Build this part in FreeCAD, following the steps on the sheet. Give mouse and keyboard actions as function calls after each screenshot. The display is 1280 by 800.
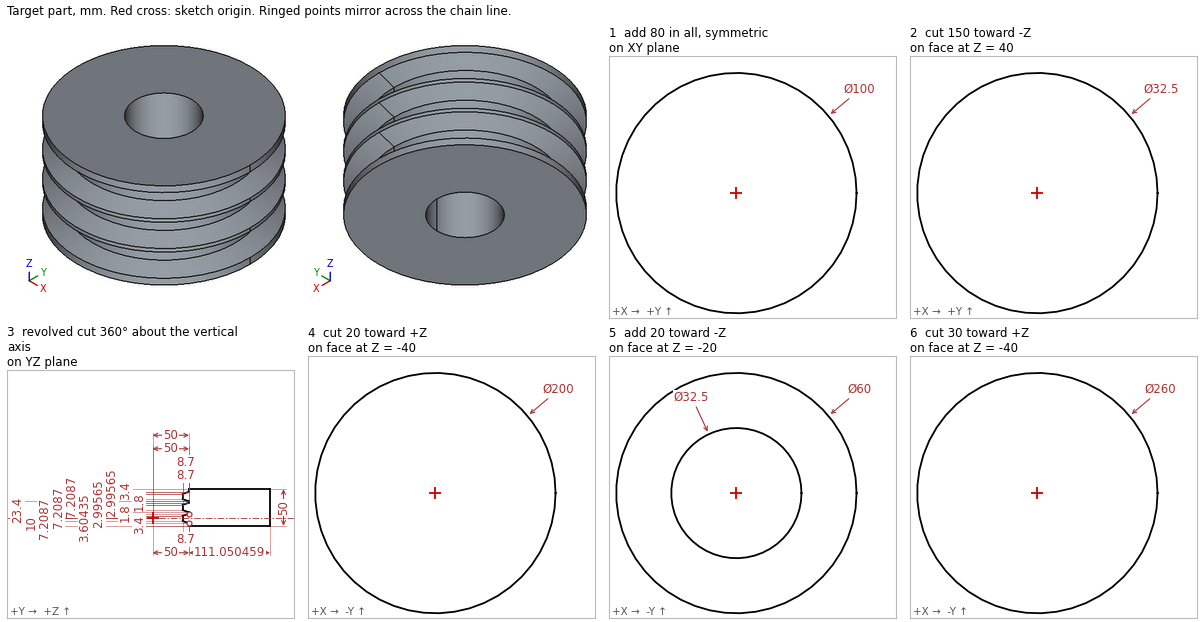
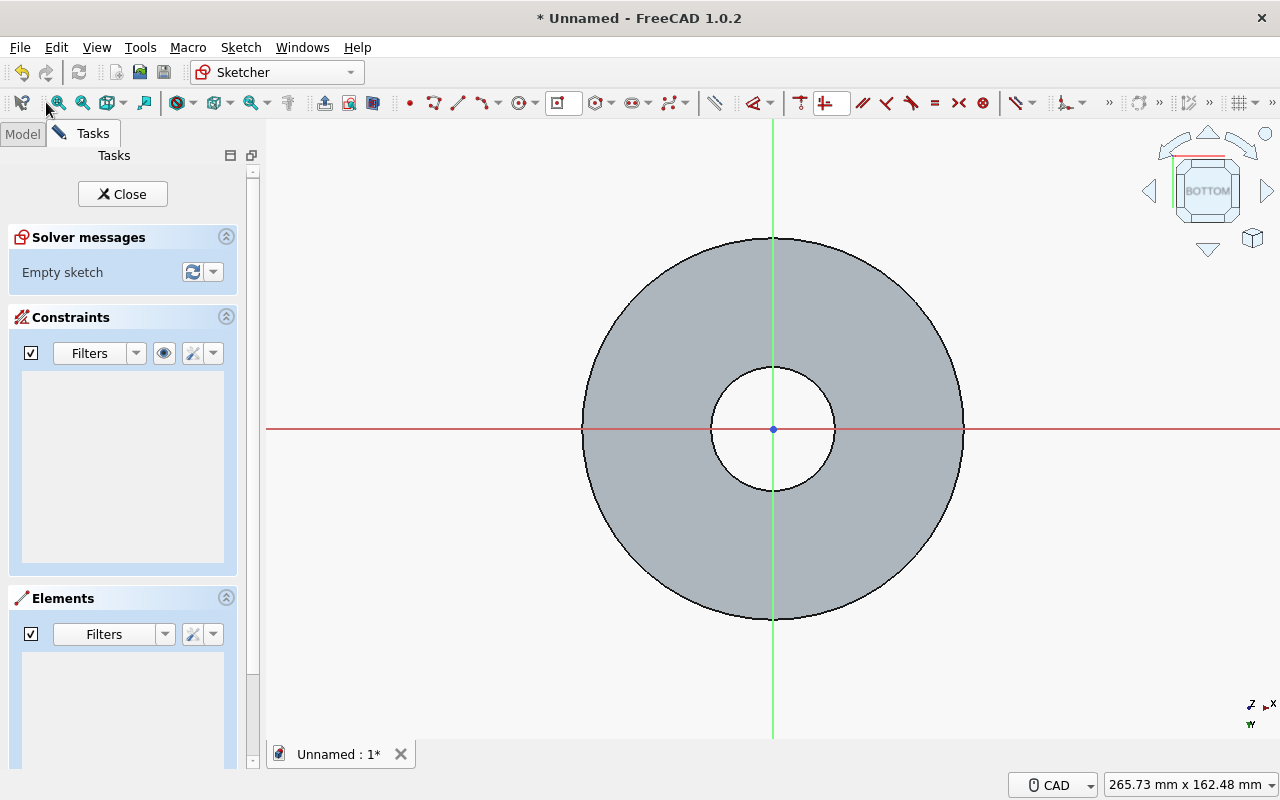
scroll(621, 429, down, 3)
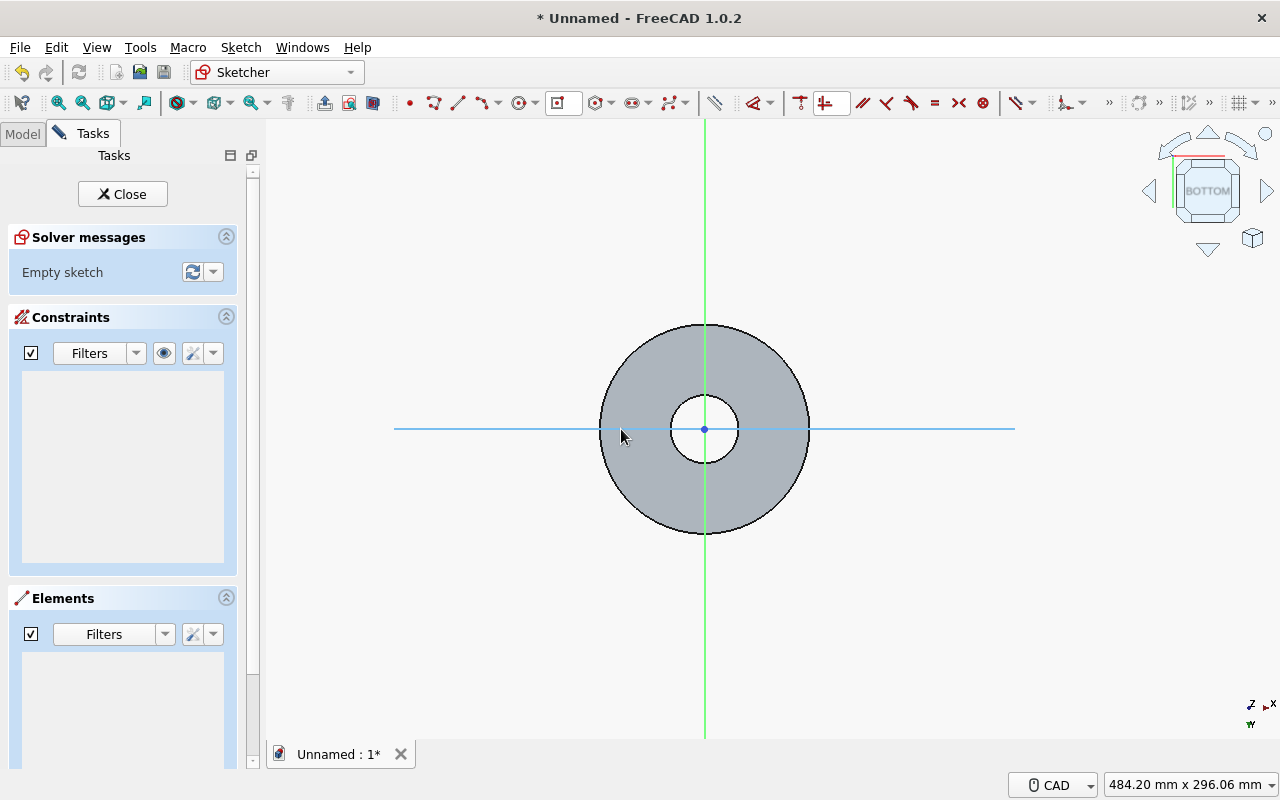
click(520, 104)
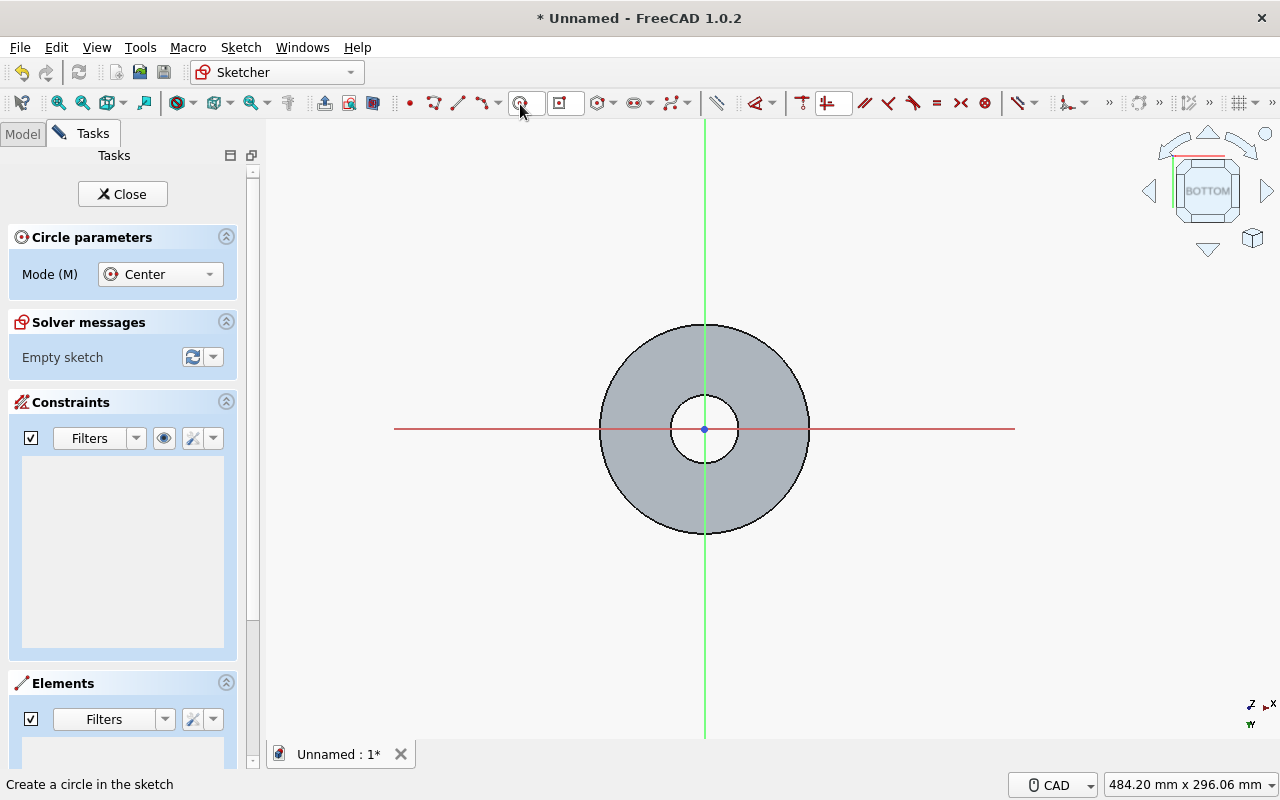
click(705, 429)
click(853, 281)
key(Escape)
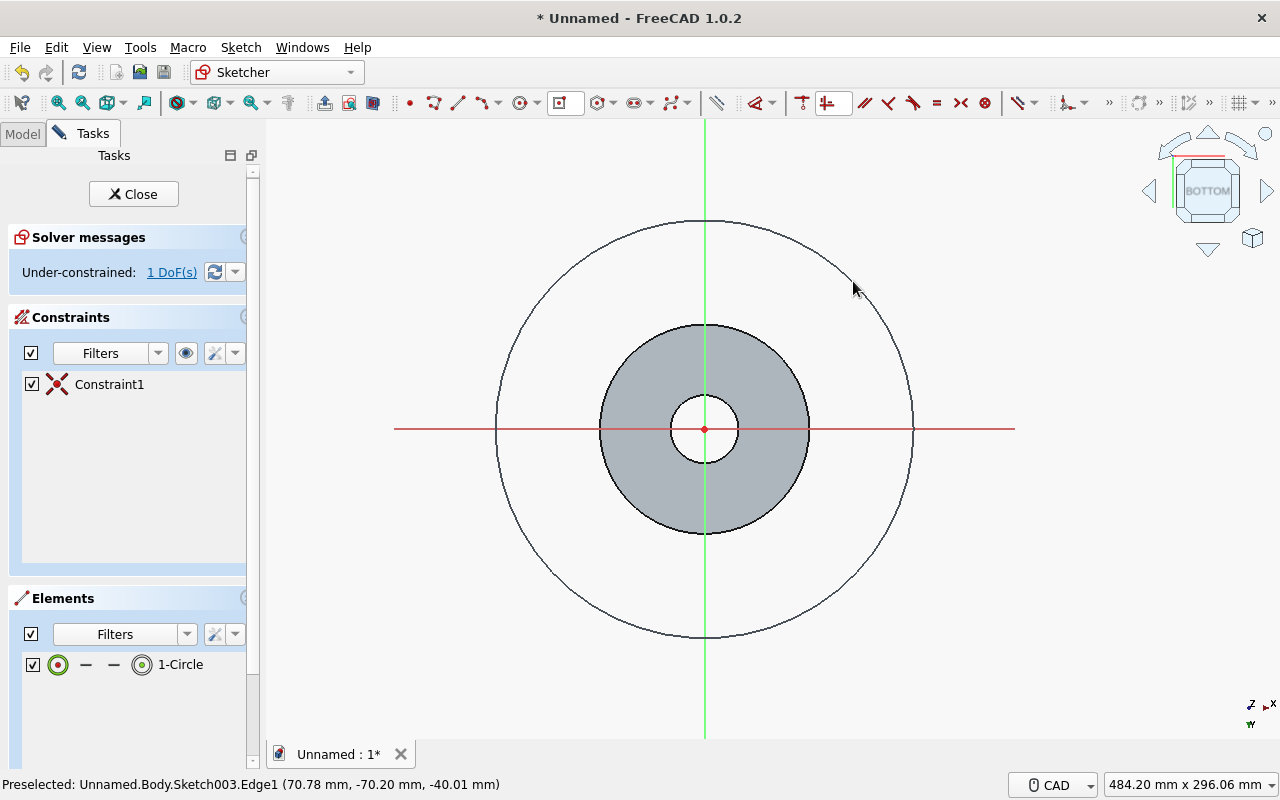
click(756, 104)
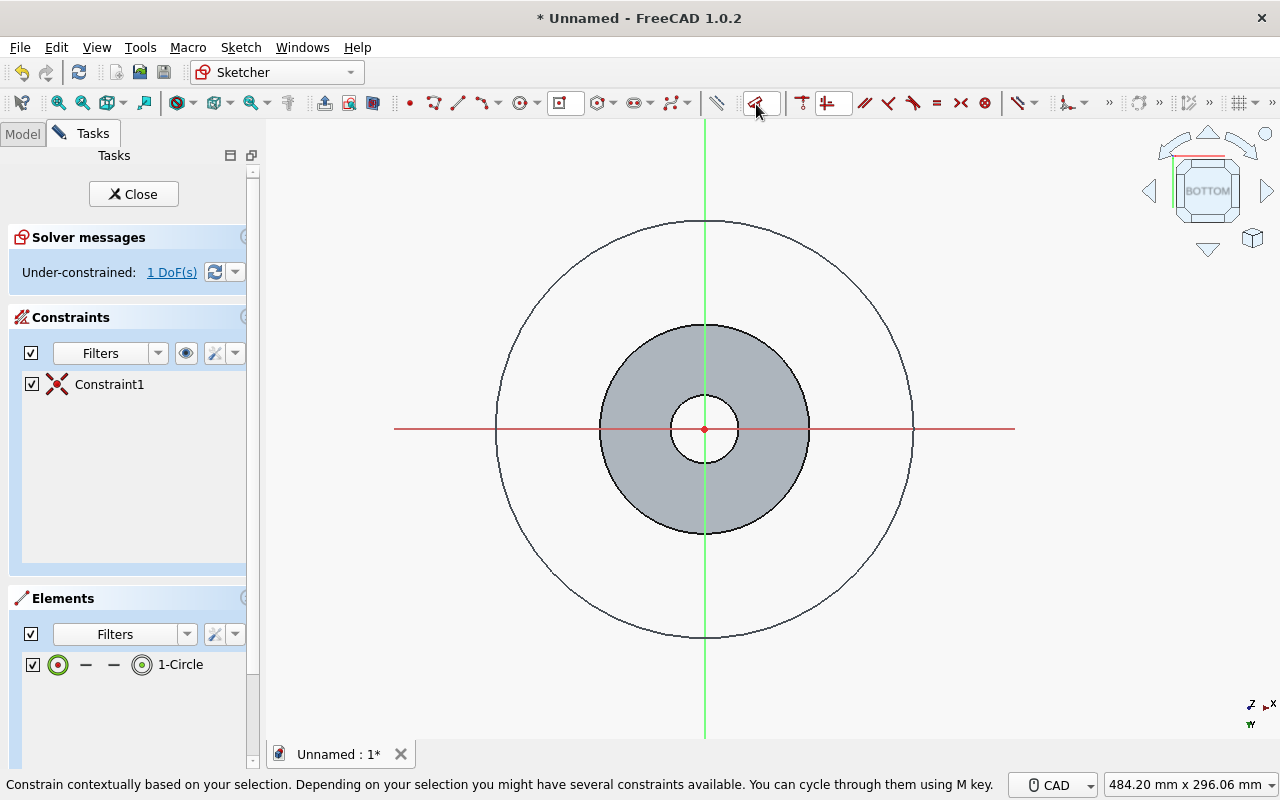
click(852, 281)
click(875, 258)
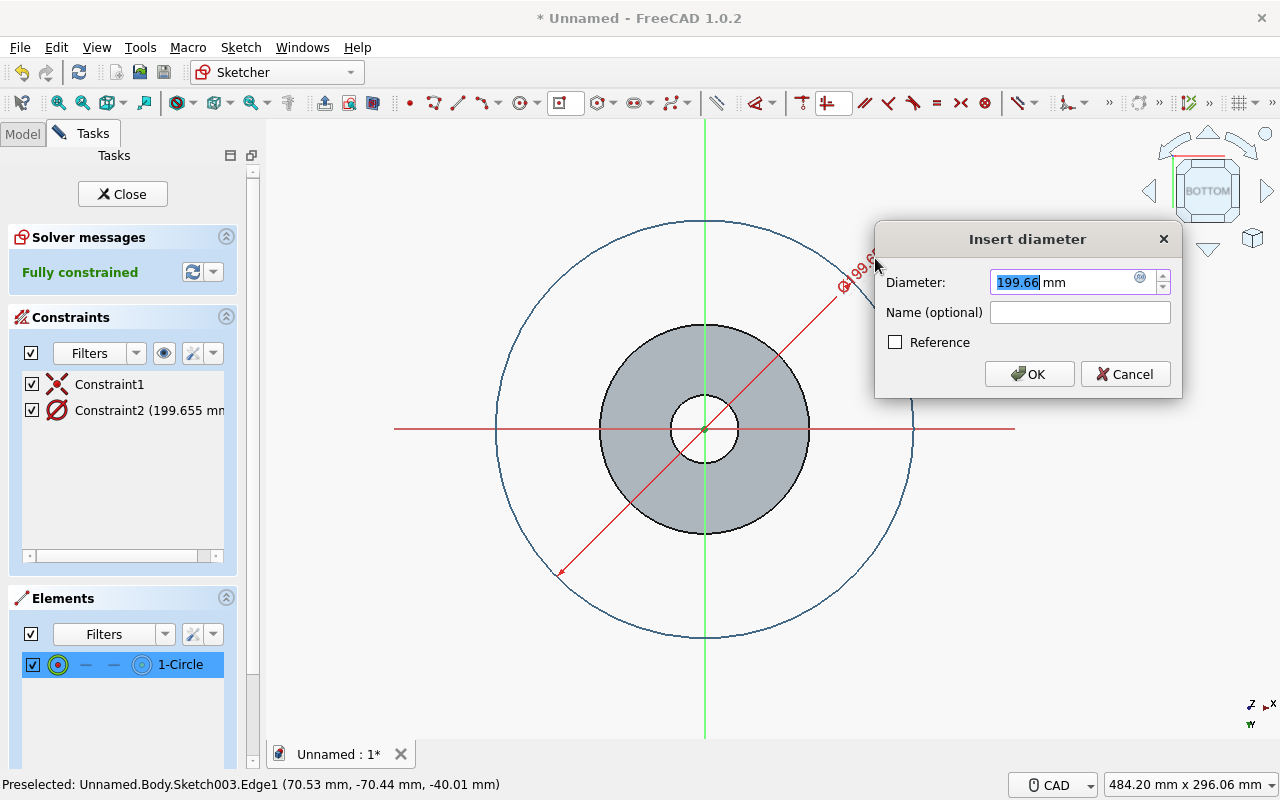
text(200)
key(Return)
key(Escape)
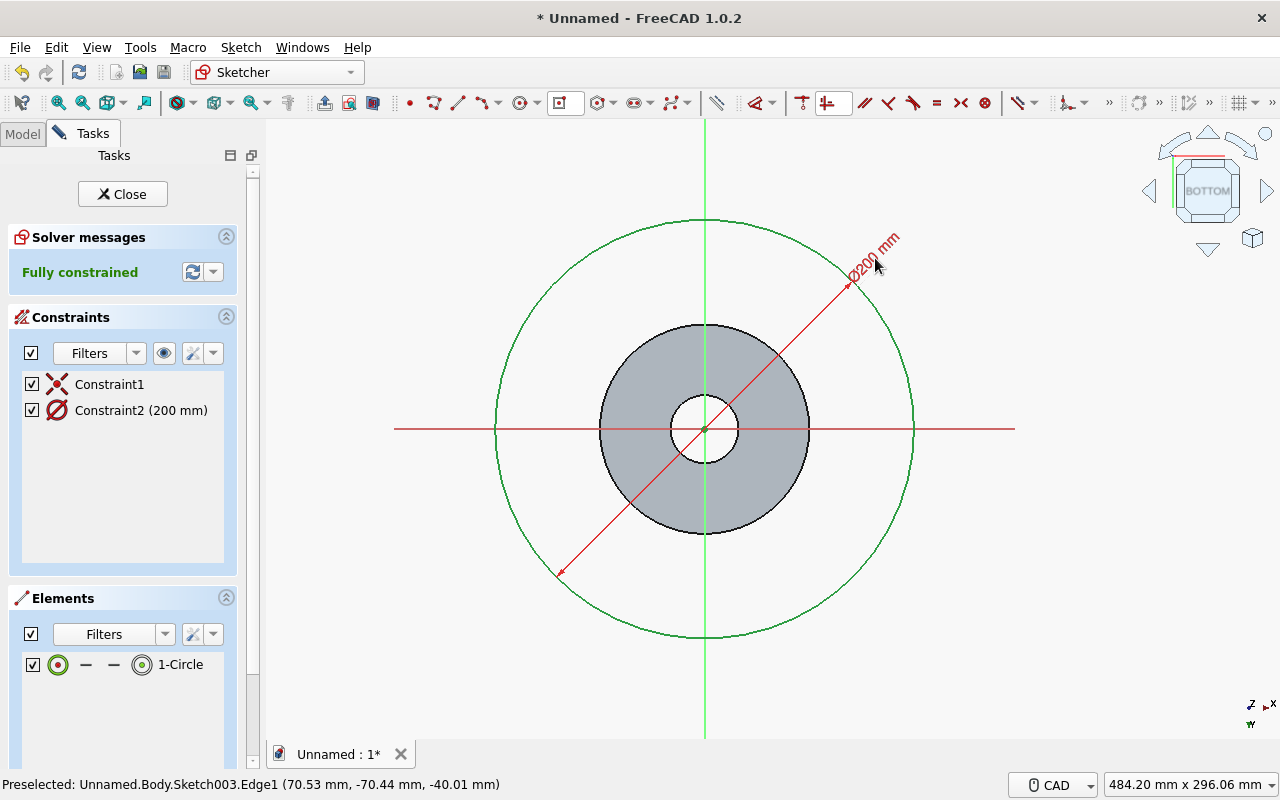
click(123, 194)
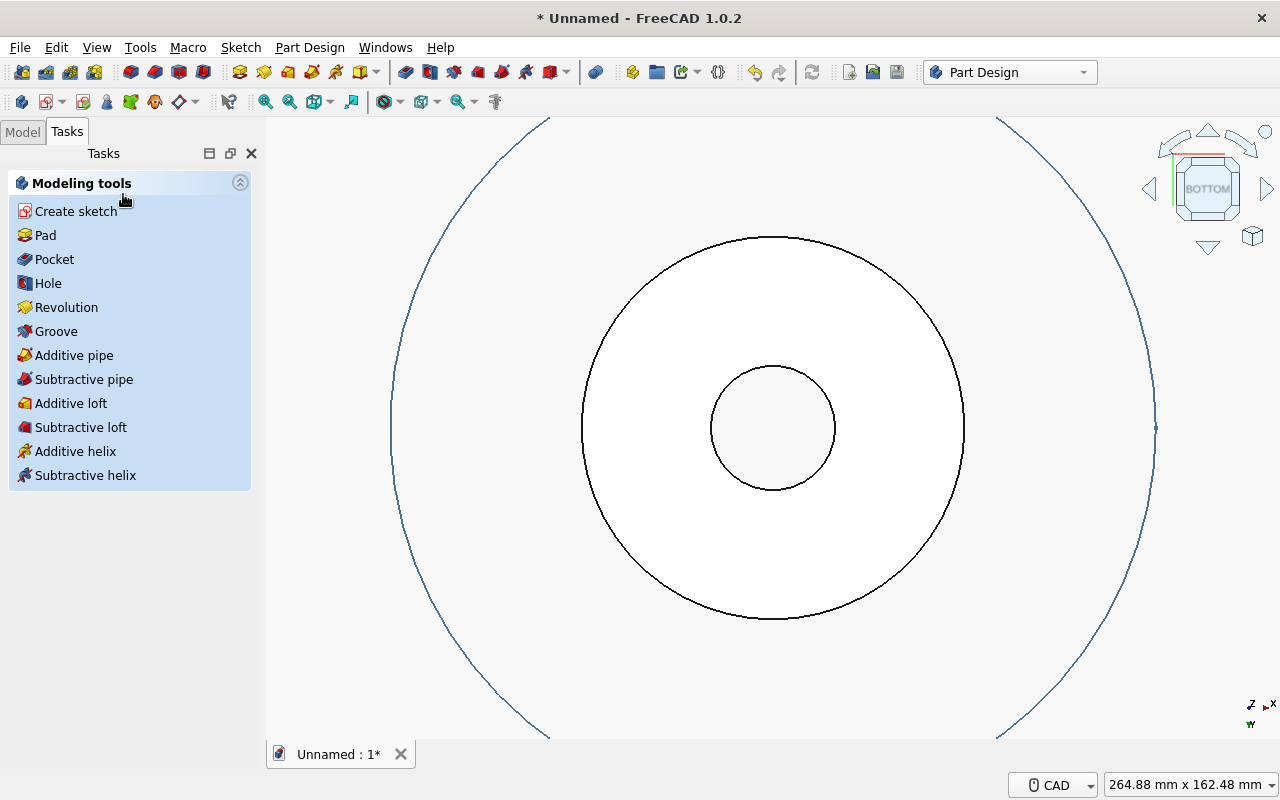
click(406, 72)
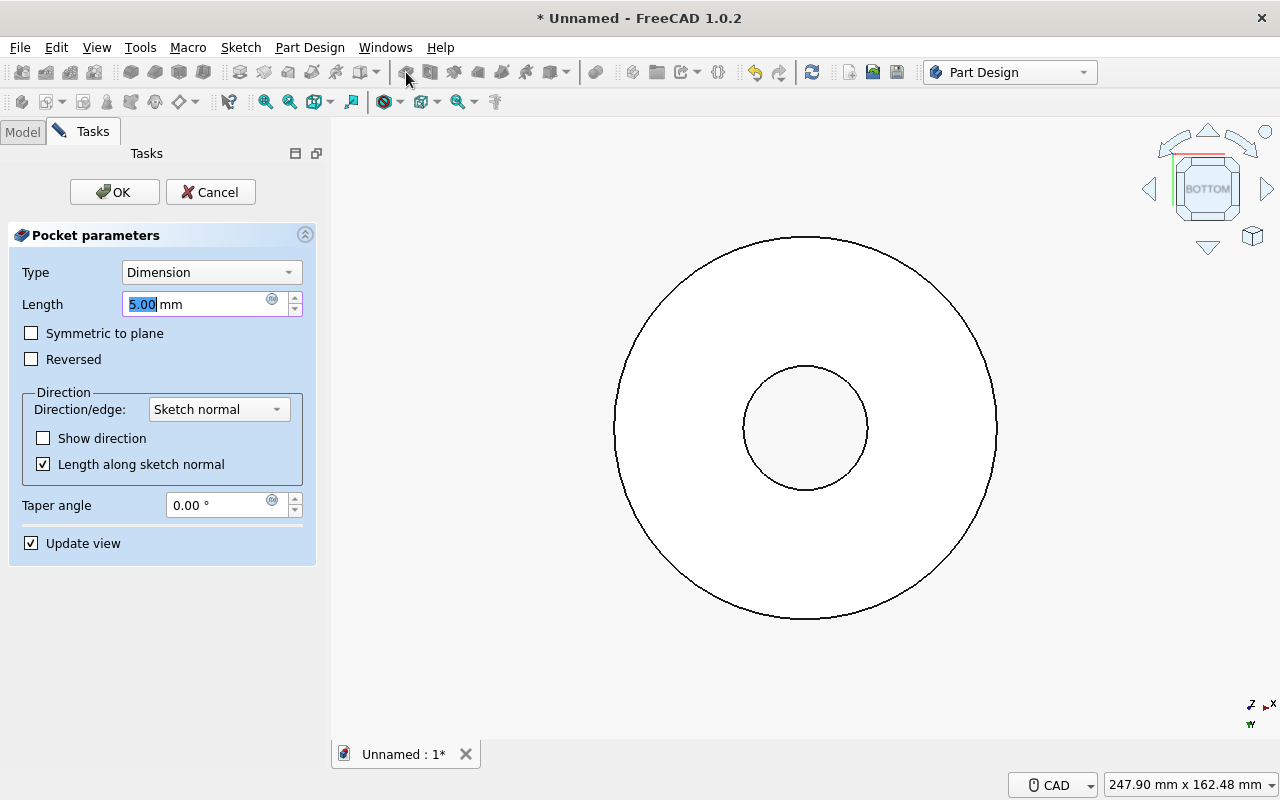
text(20)
key(Tab)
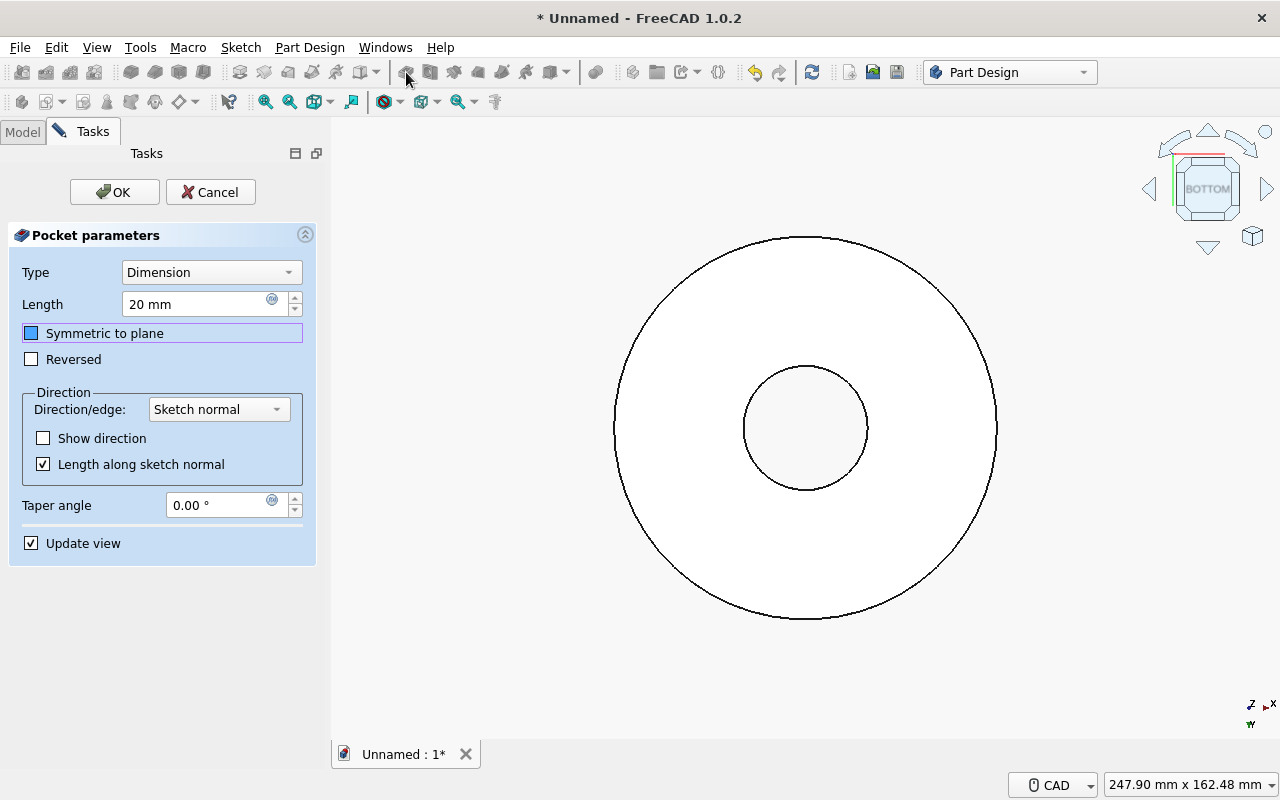
click(115, 192)